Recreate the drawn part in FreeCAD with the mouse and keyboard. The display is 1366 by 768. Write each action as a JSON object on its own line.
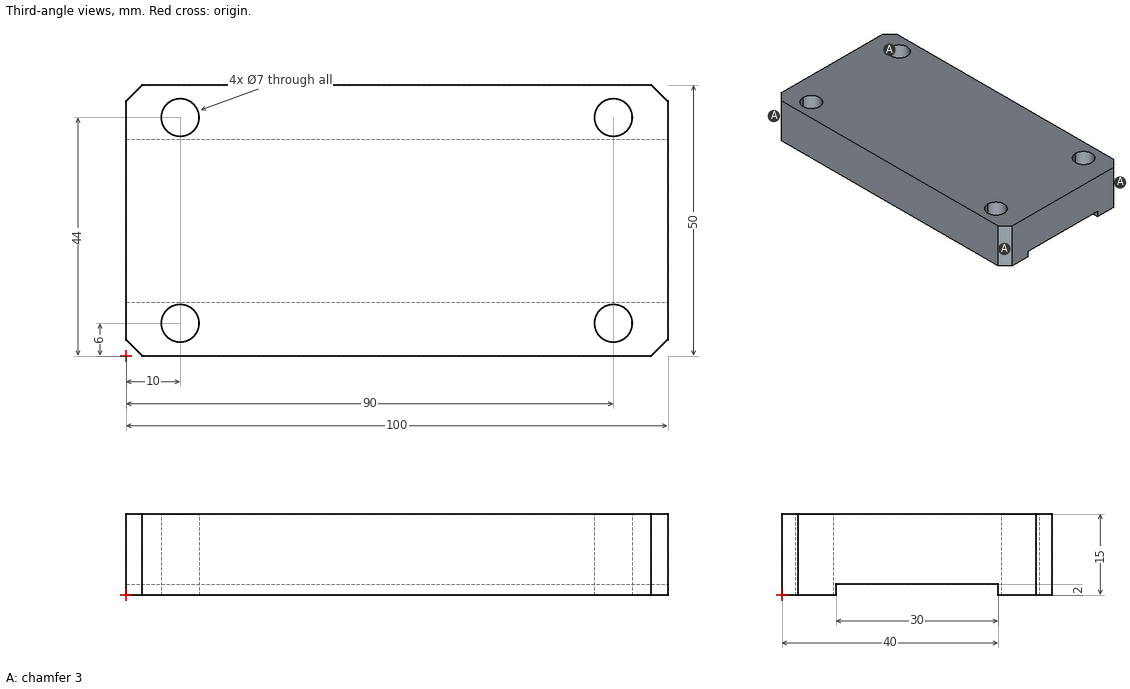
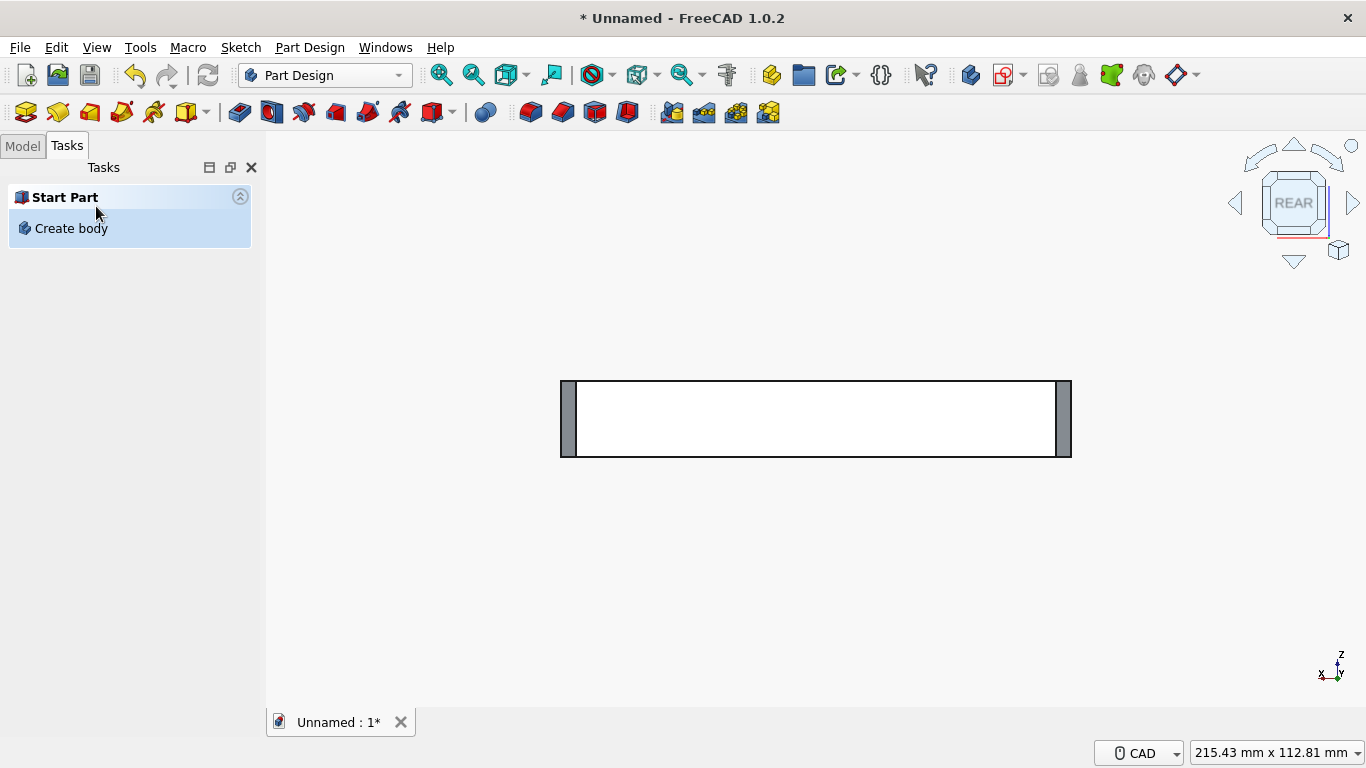
{"action": "key", "text": "6"}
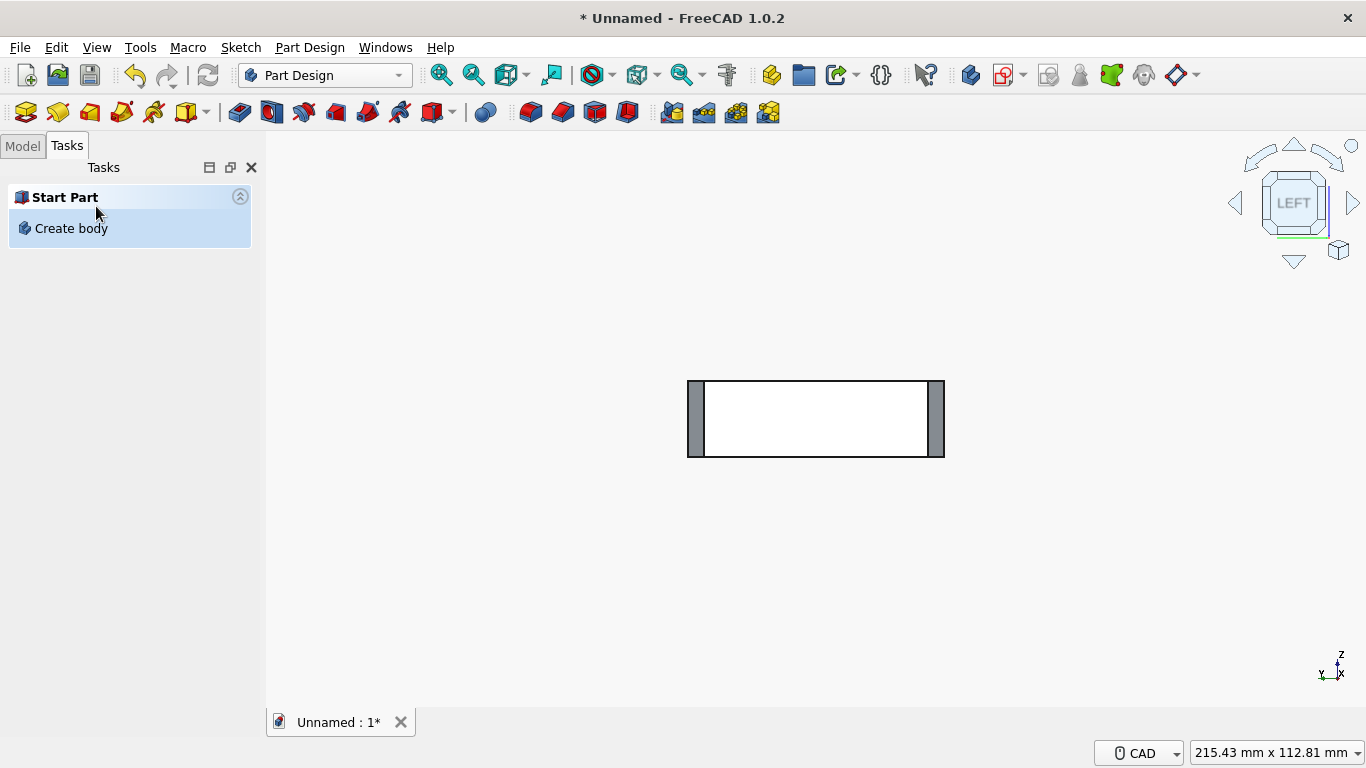
{"action": "left_click", "coordinate": [442, 76]}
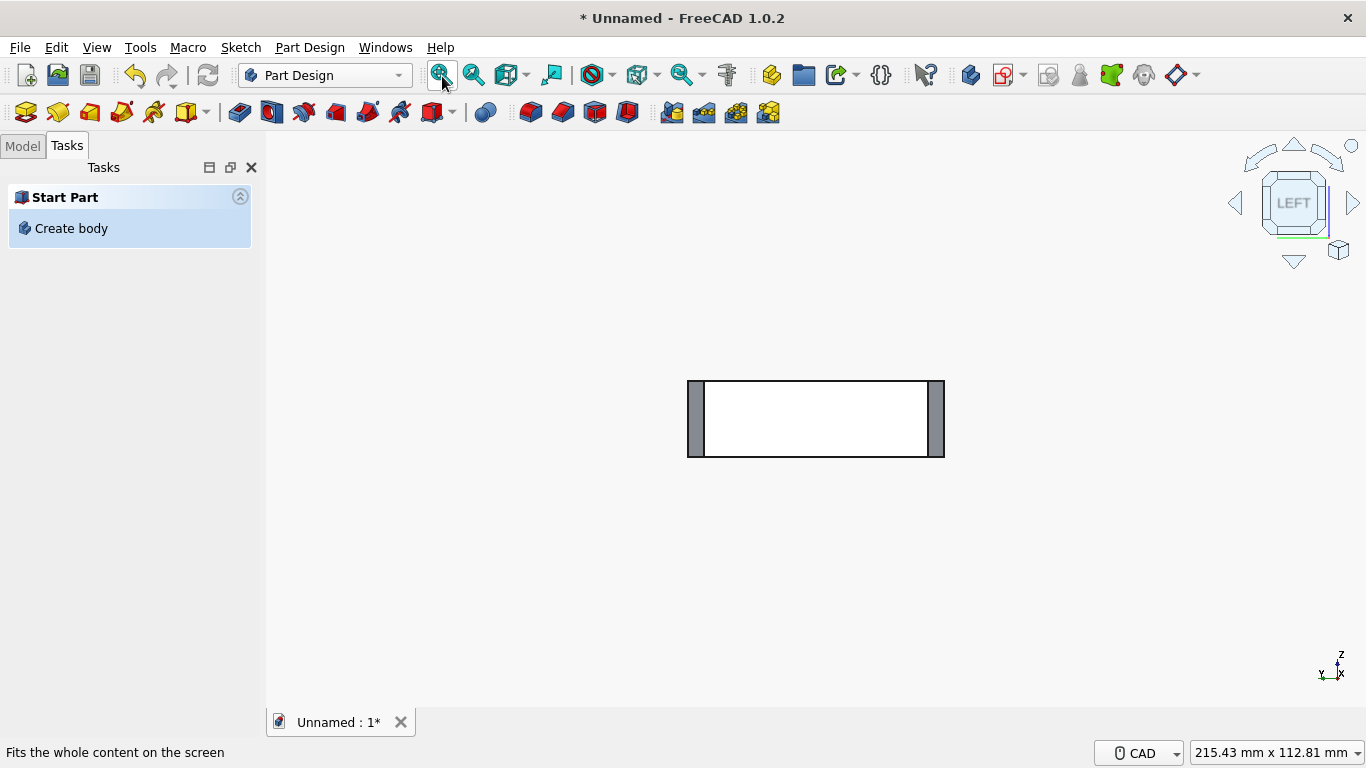
{"action": "left_click", "coordinate": [752, 418]}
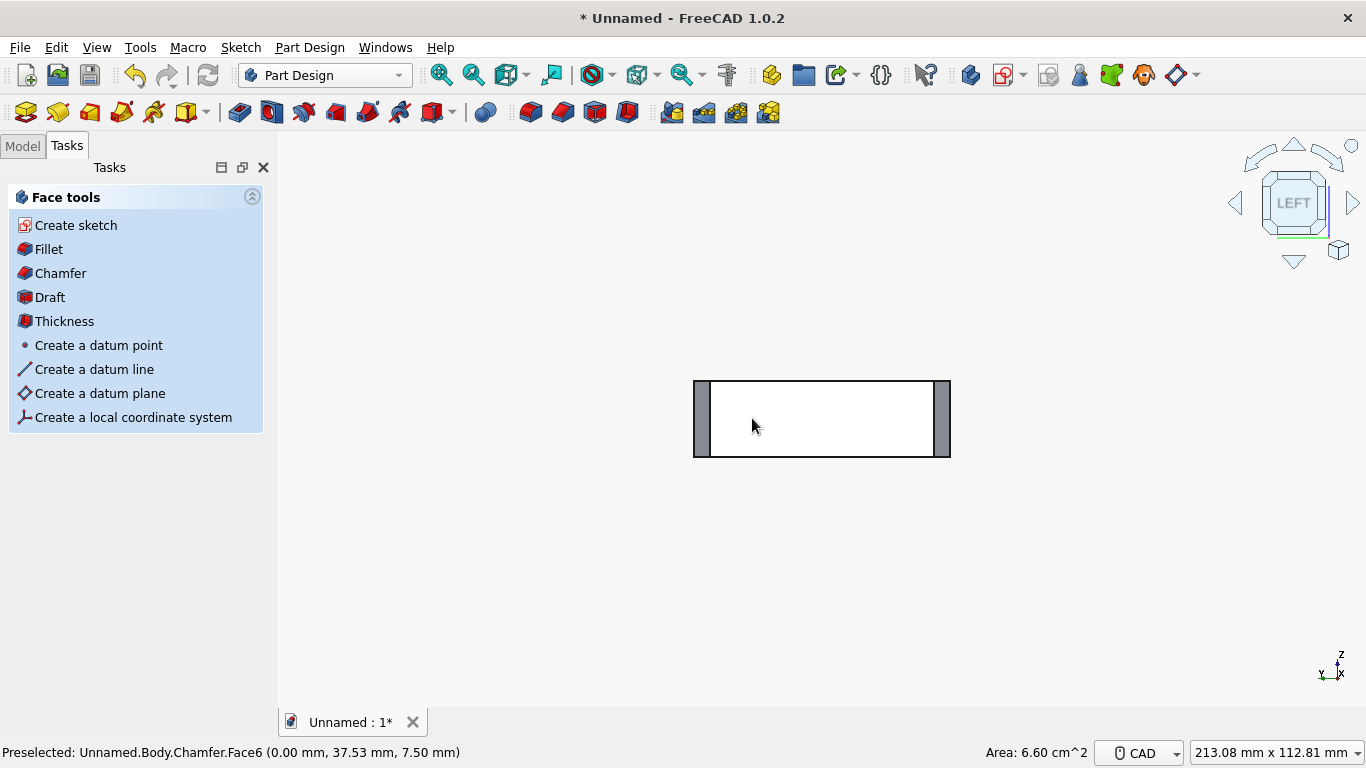
{"action": "left_click", "coordinate": [1004, 76]}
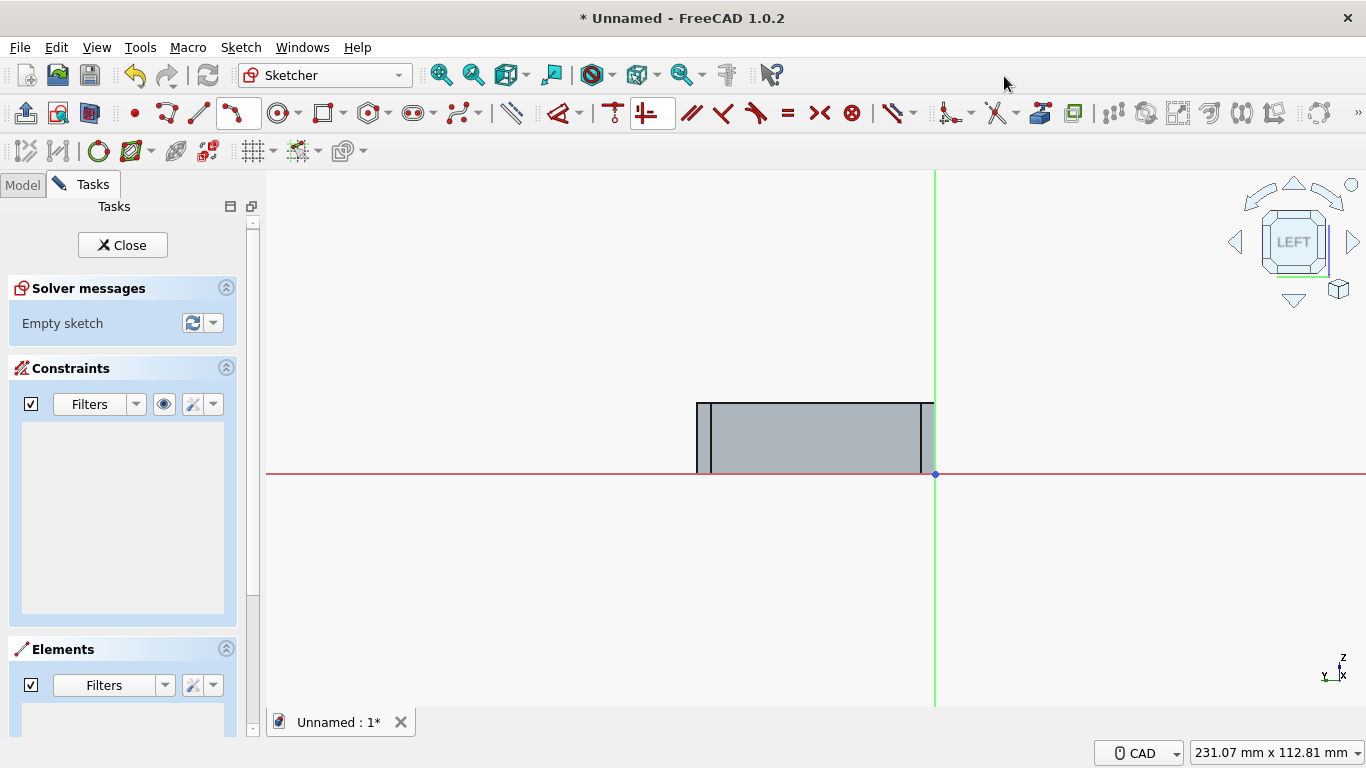
{"action": "scroll", "coordinate": [880, 483], "scroll_direction": "up", "scroll_amount": 6}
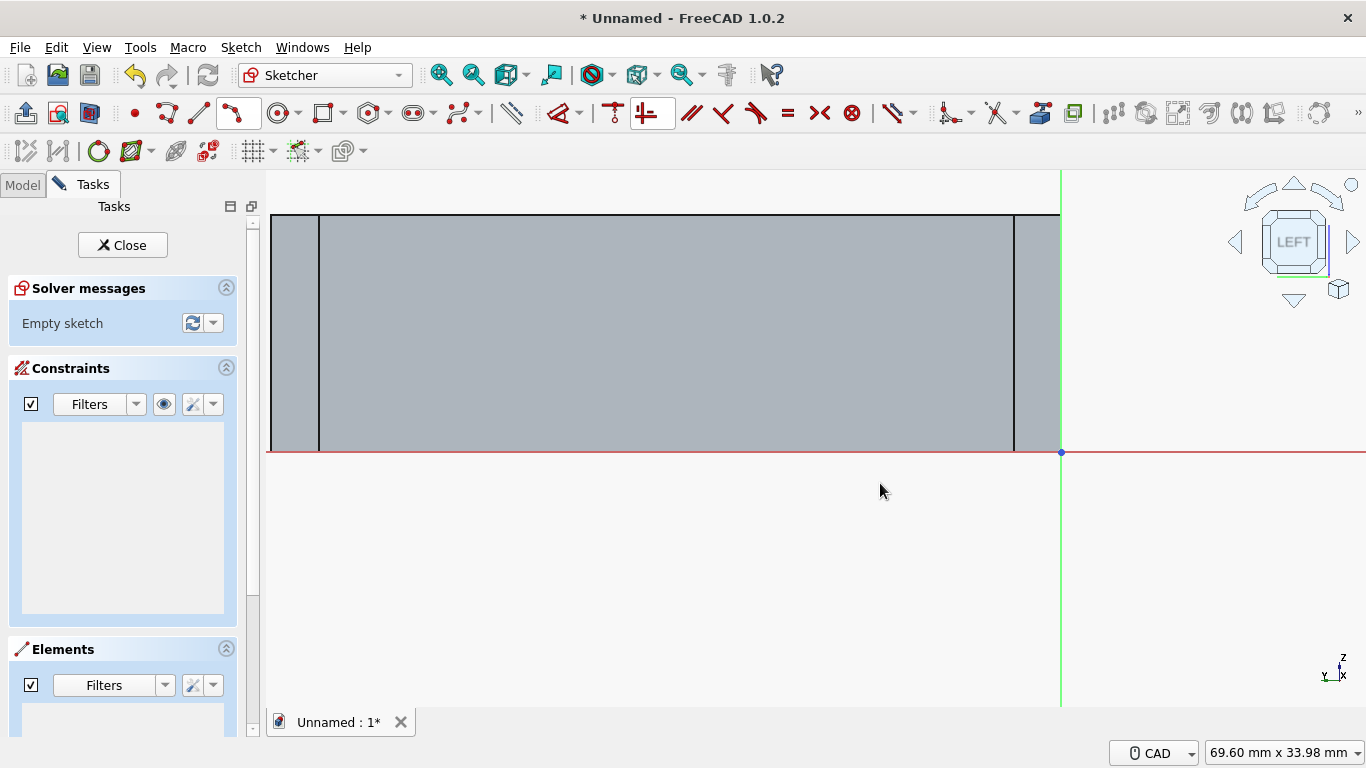
{"action": "key", "text": "g r"}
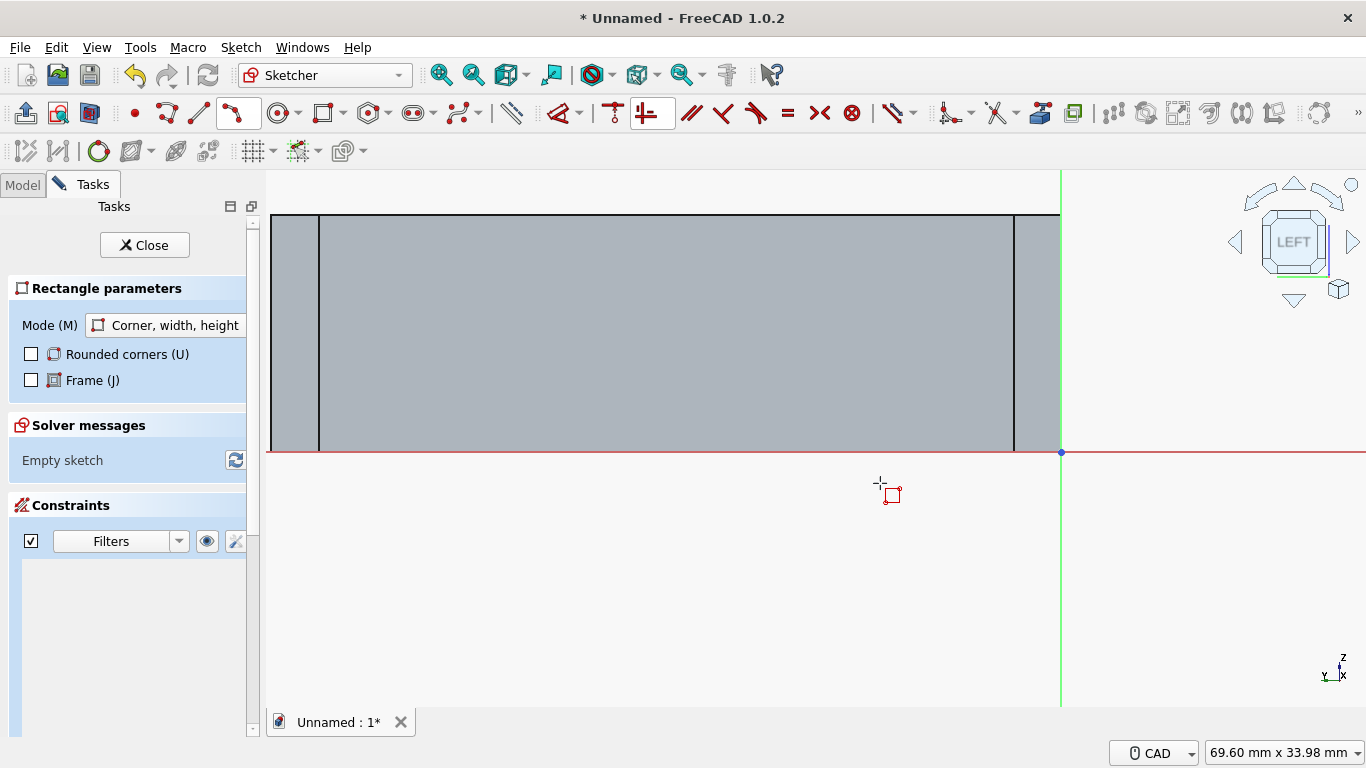
{"action": "left_click", "coordinate": [429, 421]}
{"action": "left_click", "coordinate": [903, 452]}
{"action": "key", "text": "Escape"}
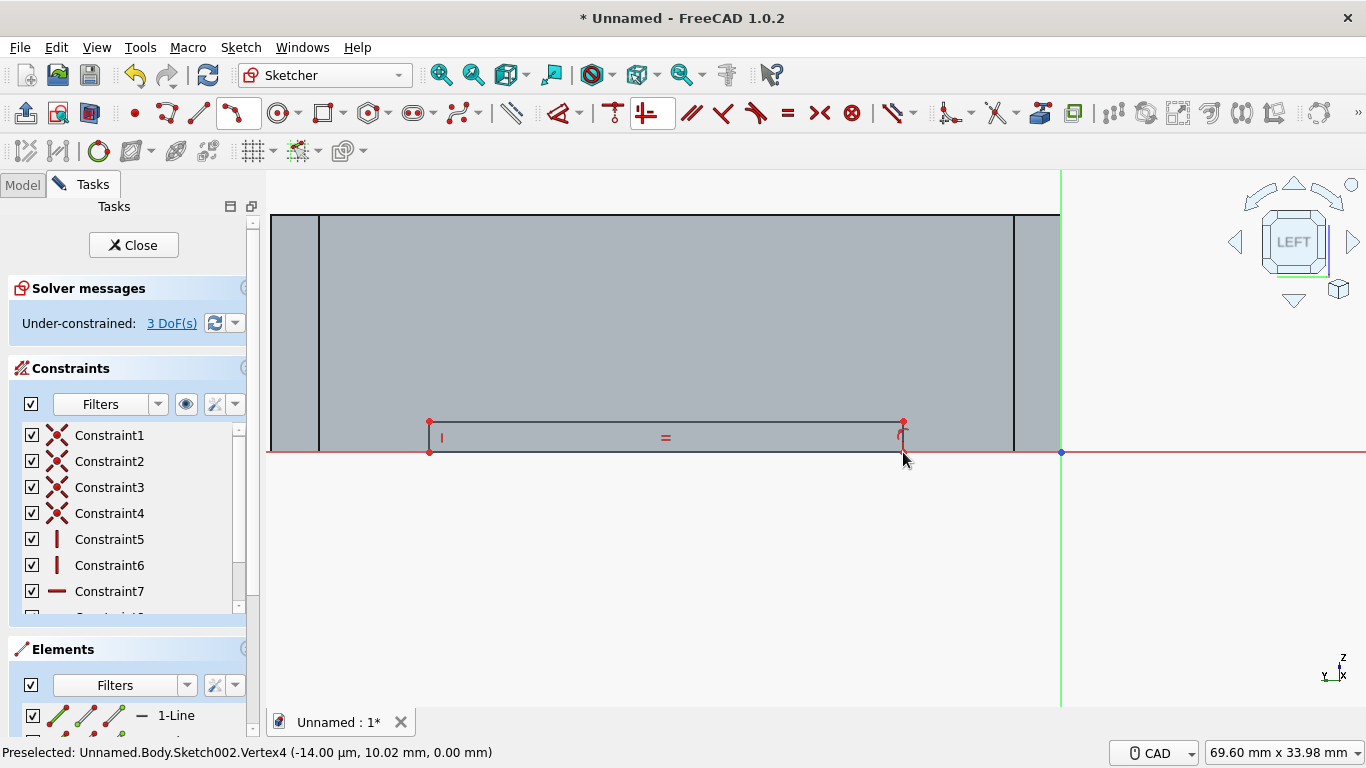
{"action": "left_click", "coordinate": [558, 114]}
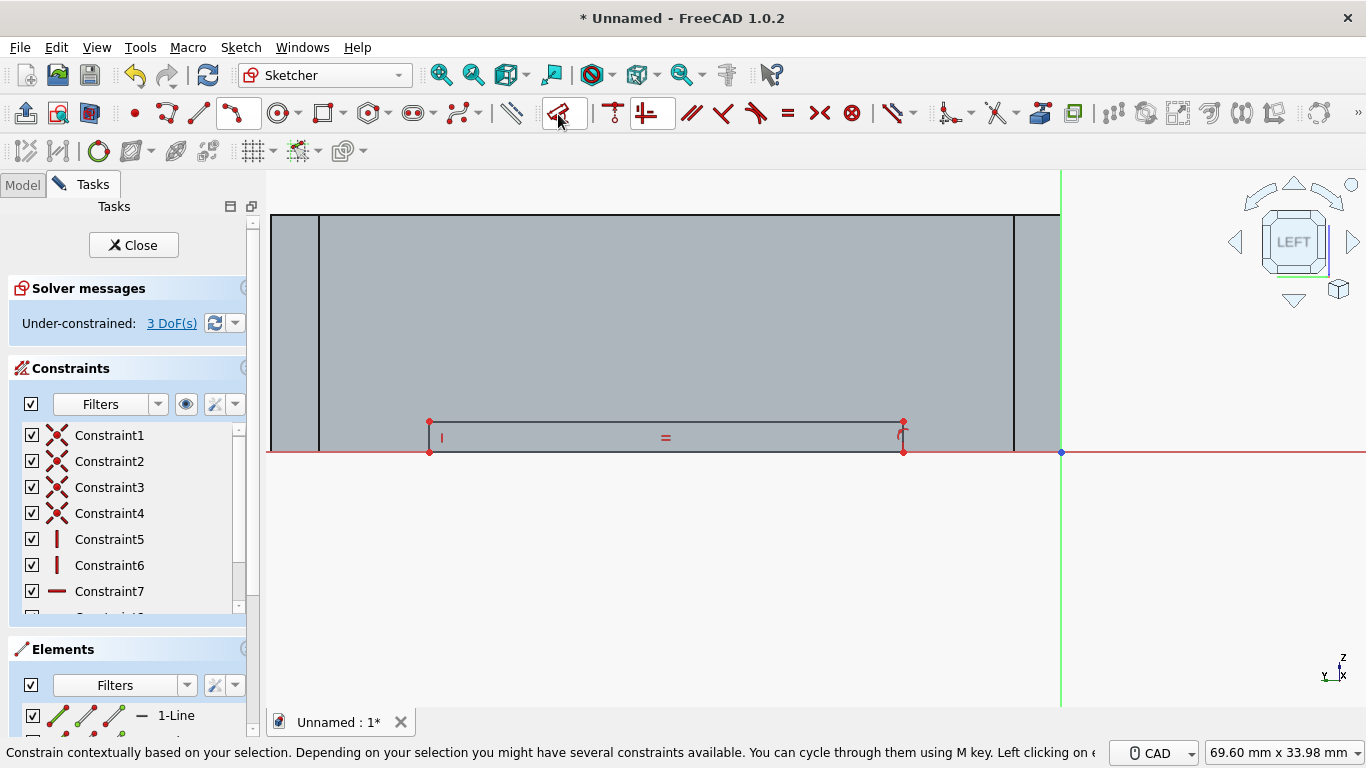
{"action": "scroll", "coordinate": [429, 431], "scroll_direction": "up", "scroll_amount": 3}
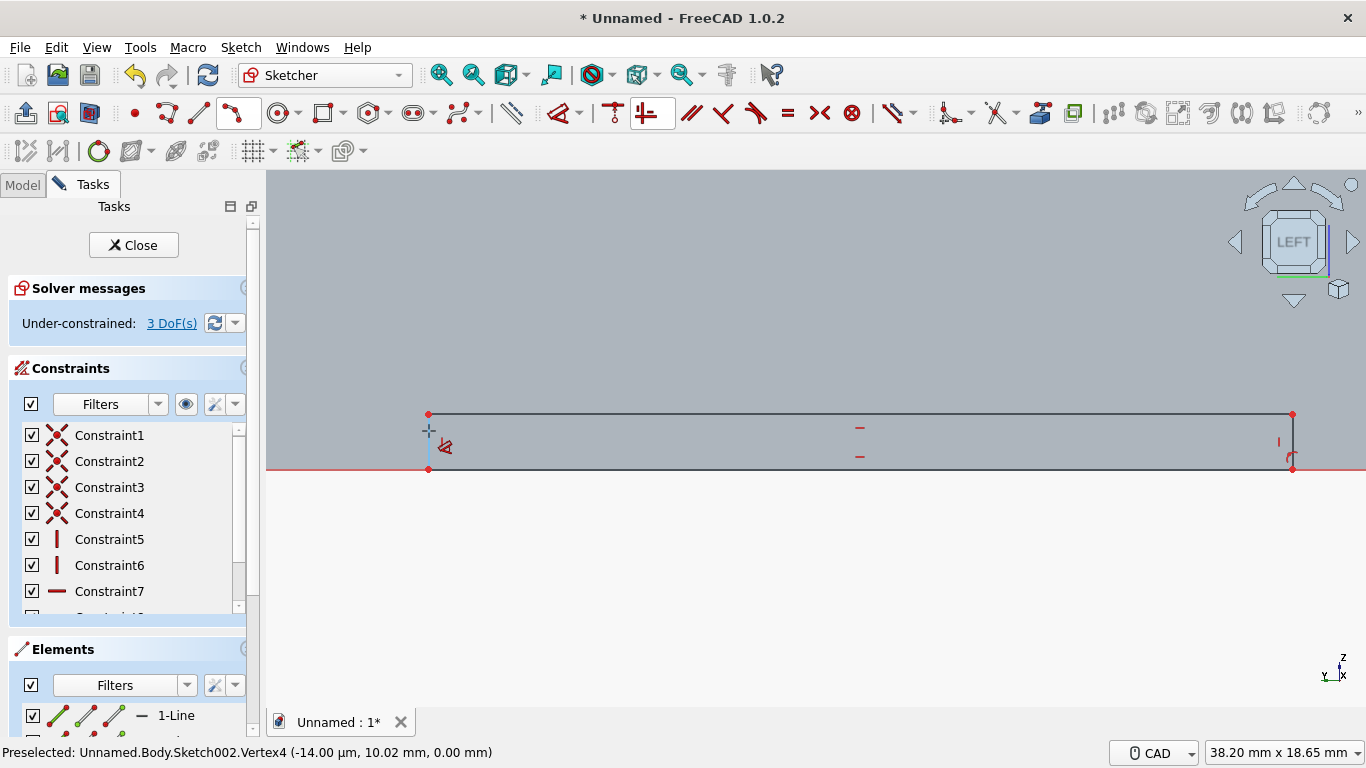
{"action": "left_click", "coordinate": [429, 431]}
{"action": "left_click", "coordinate": [395, 442]}